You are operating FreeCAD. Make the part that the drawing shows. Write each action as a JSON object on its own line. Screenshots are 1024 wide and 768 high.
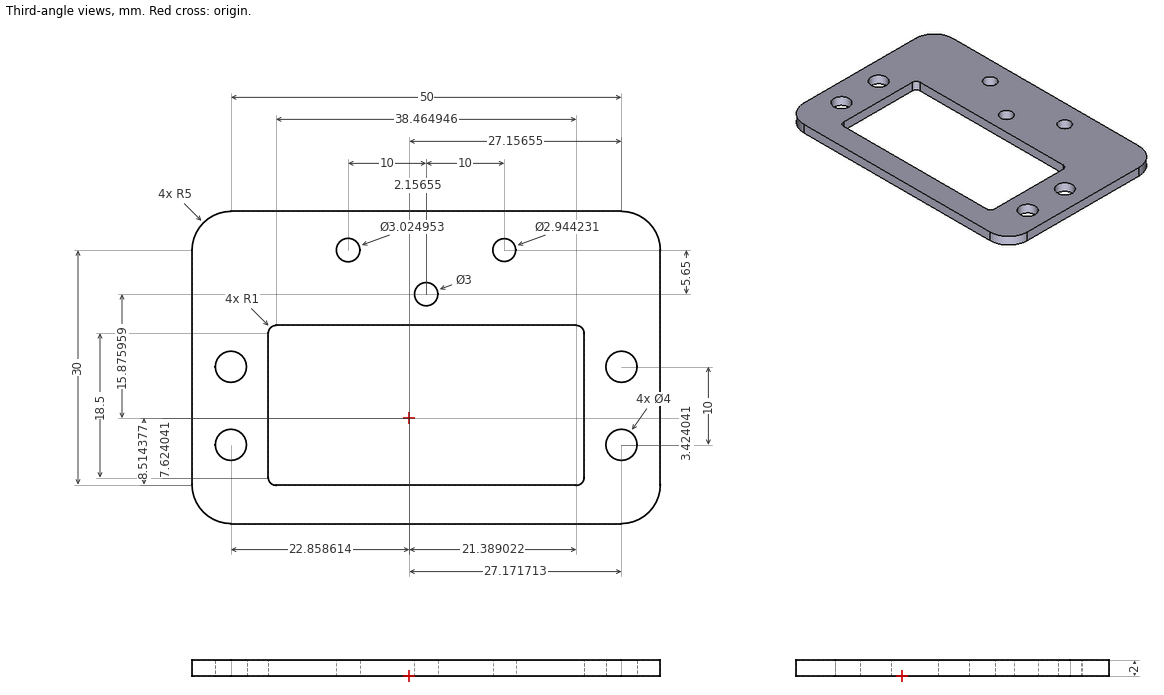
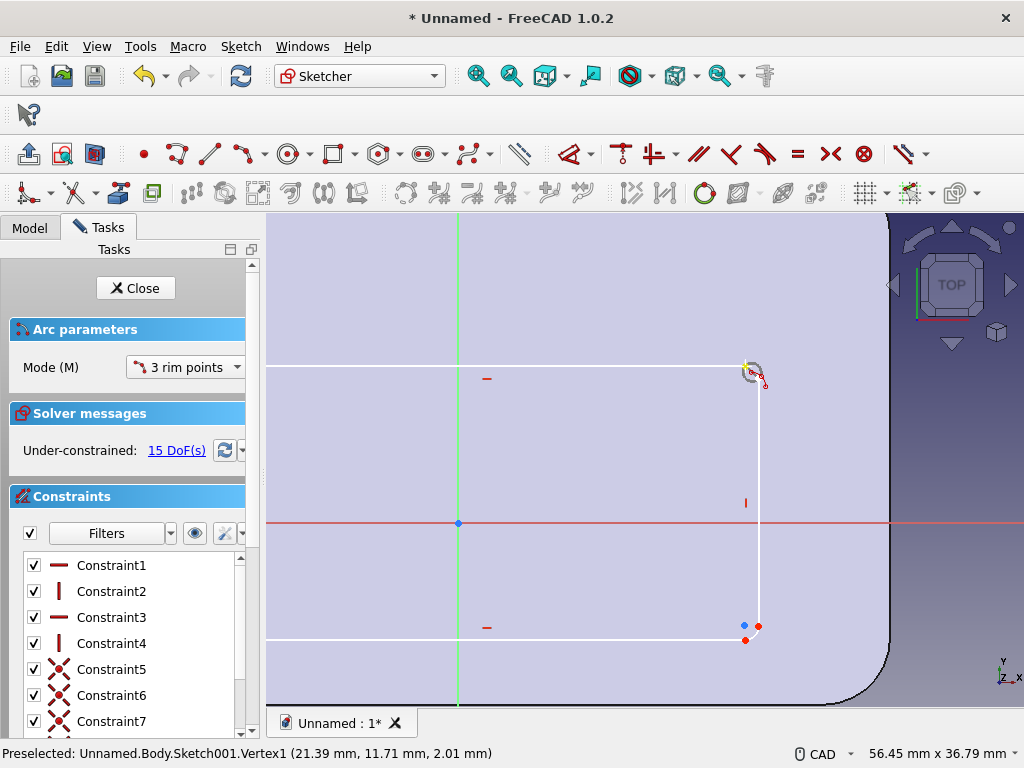
{"action": "scroll", "coordinate": [755, 368], "scroll_direction": "up", "scroll_amount": 7}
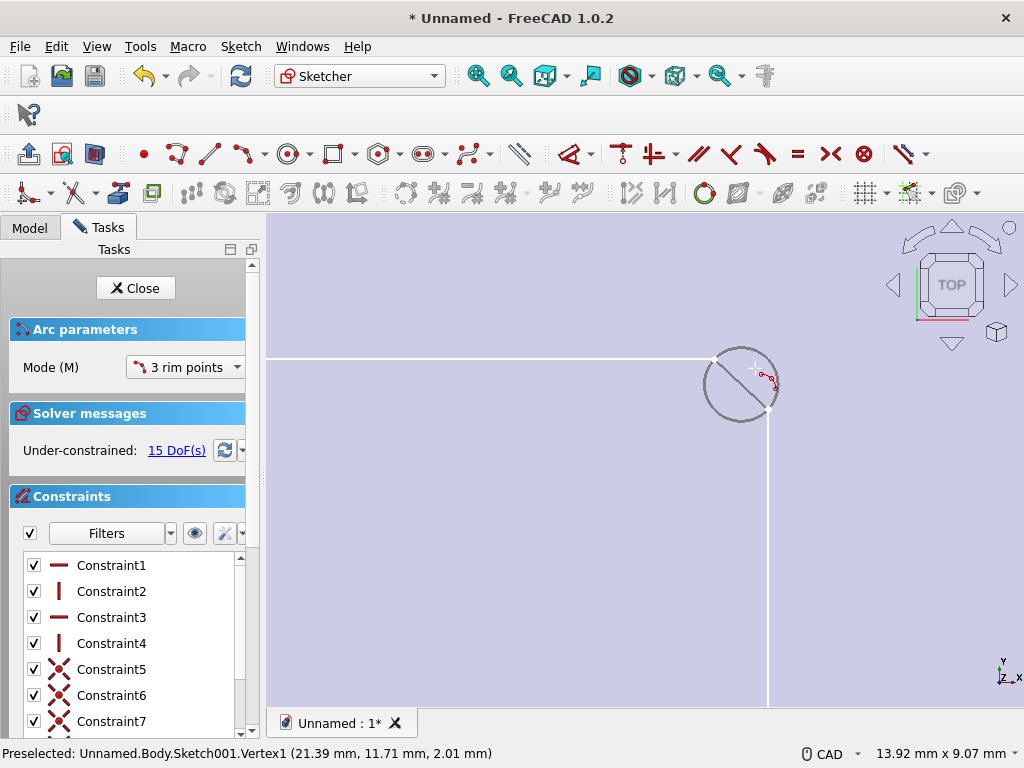
{"action": "left_click", "coordinate": [753, 366]}
{"action": "key", "text": "Escape"}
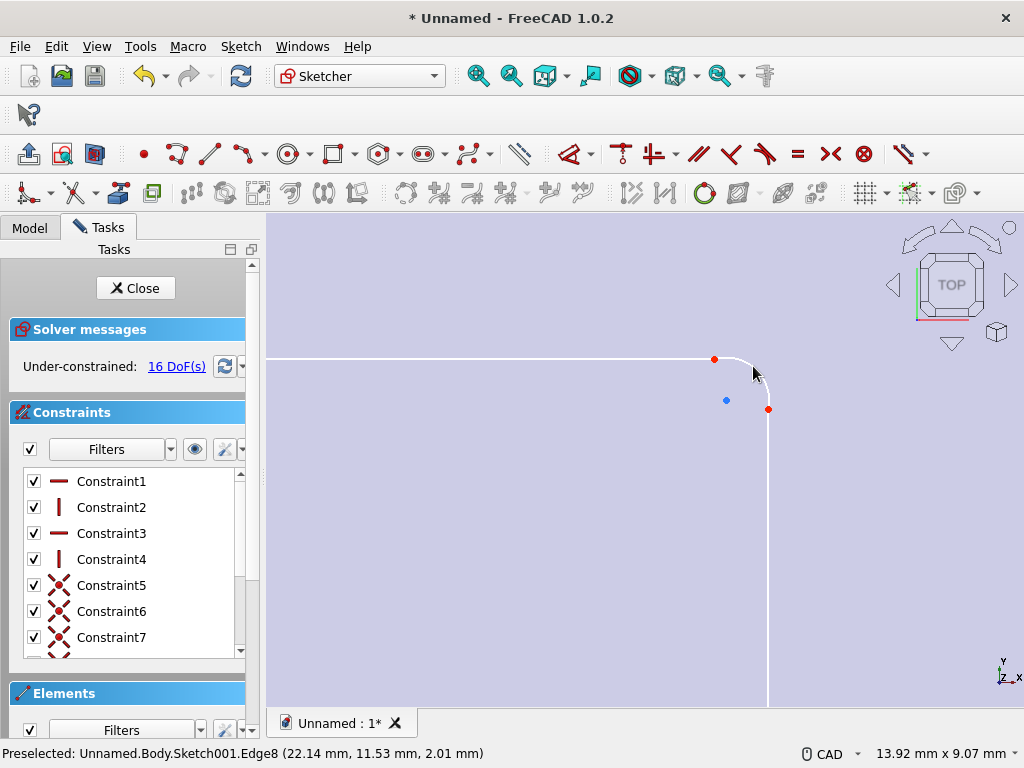
{"action": "scroll", "coordinate": [757, 371], "scroll_direction": "down", "scroll_amount": 9}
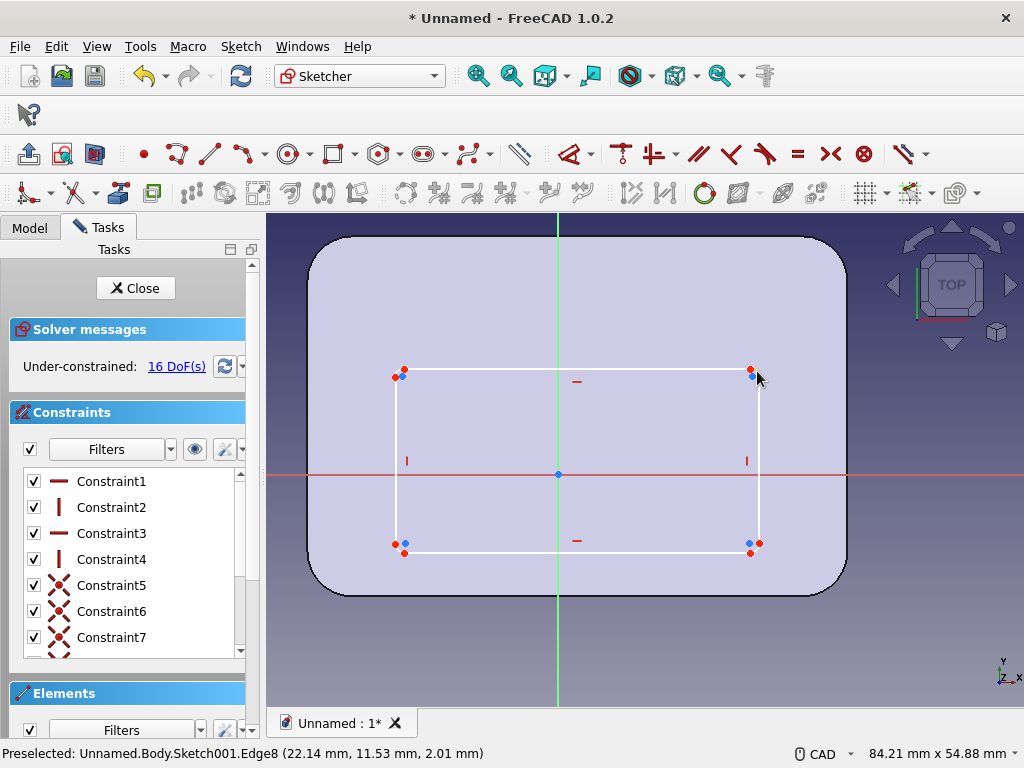
{"action": "left_click", "coordinate": [681, 369]}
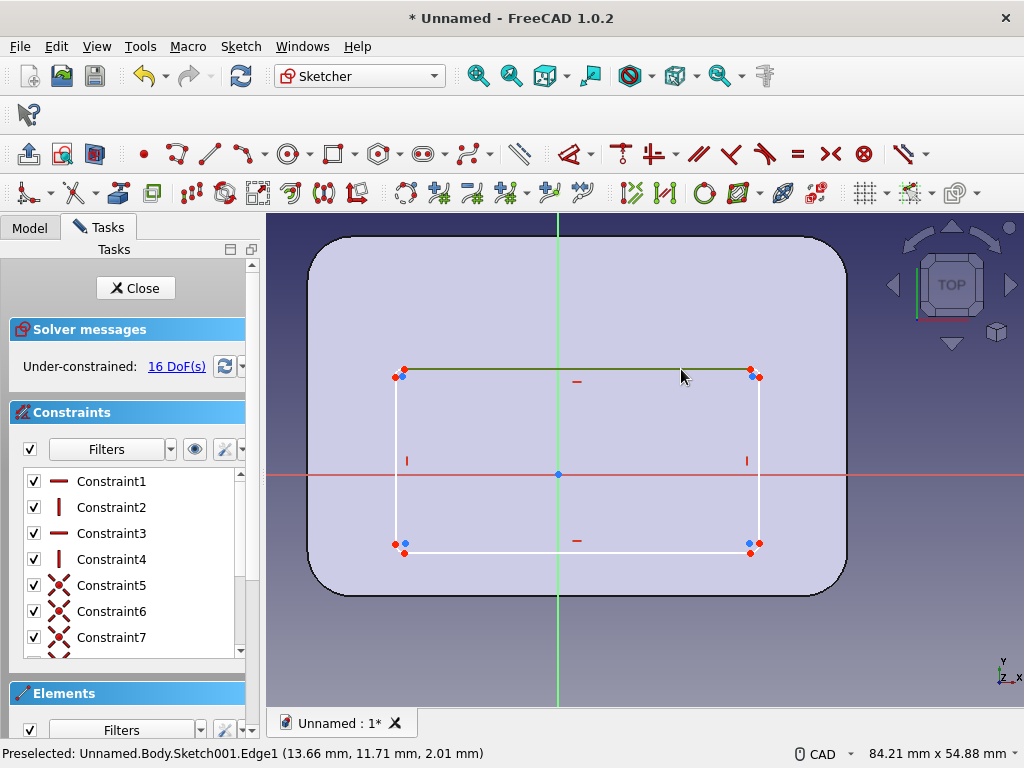
{"action": "scroll", "coordinate": [398, 371], "scroll_direction": "up", "scroll_amount": 4}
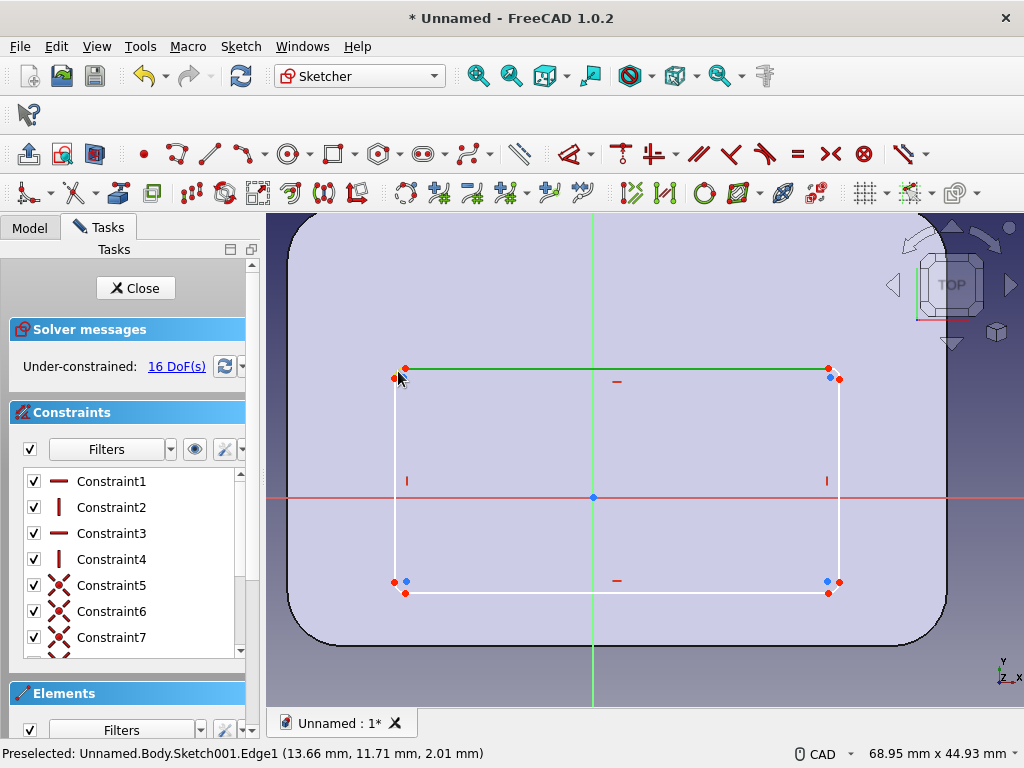
{"action": "left_click", "coordinate": [397, 370]}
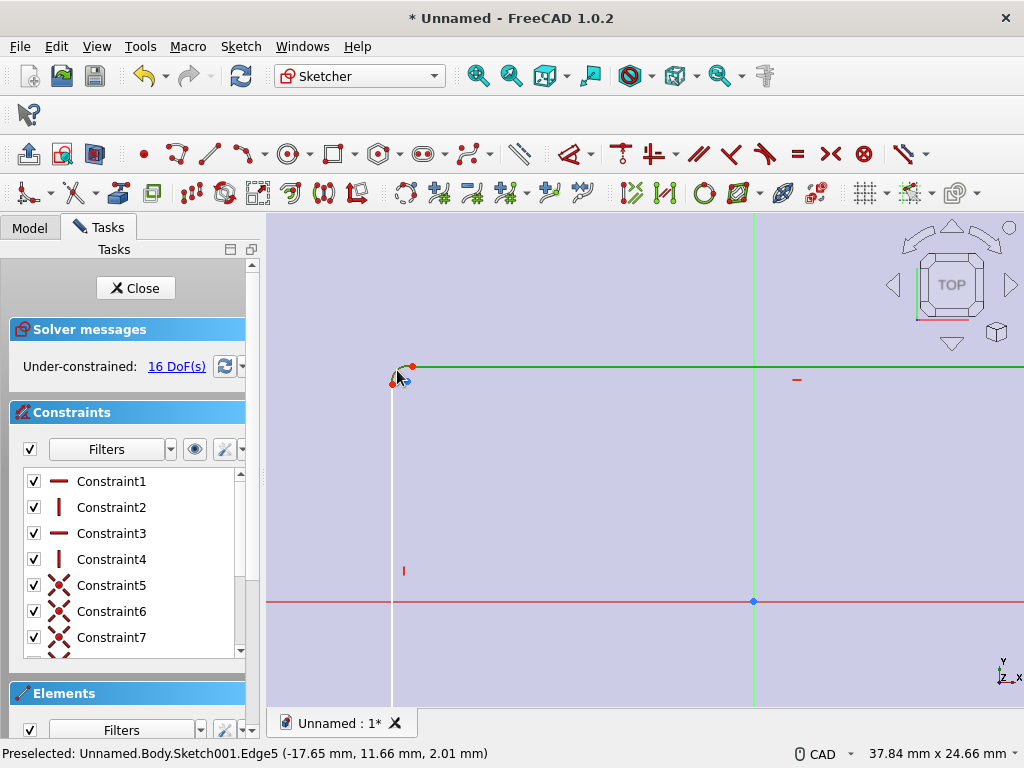
{"action": "left_click", "coordinate": [765, 154]}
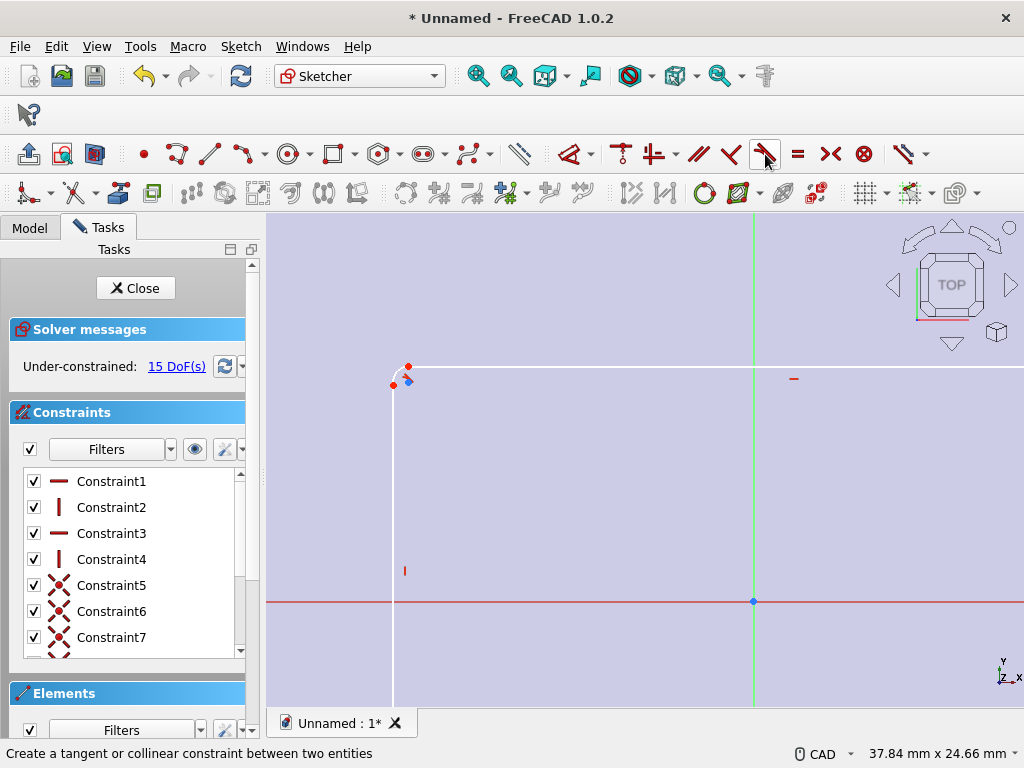
{"action": "left_click", "coordinate": [640, 367]}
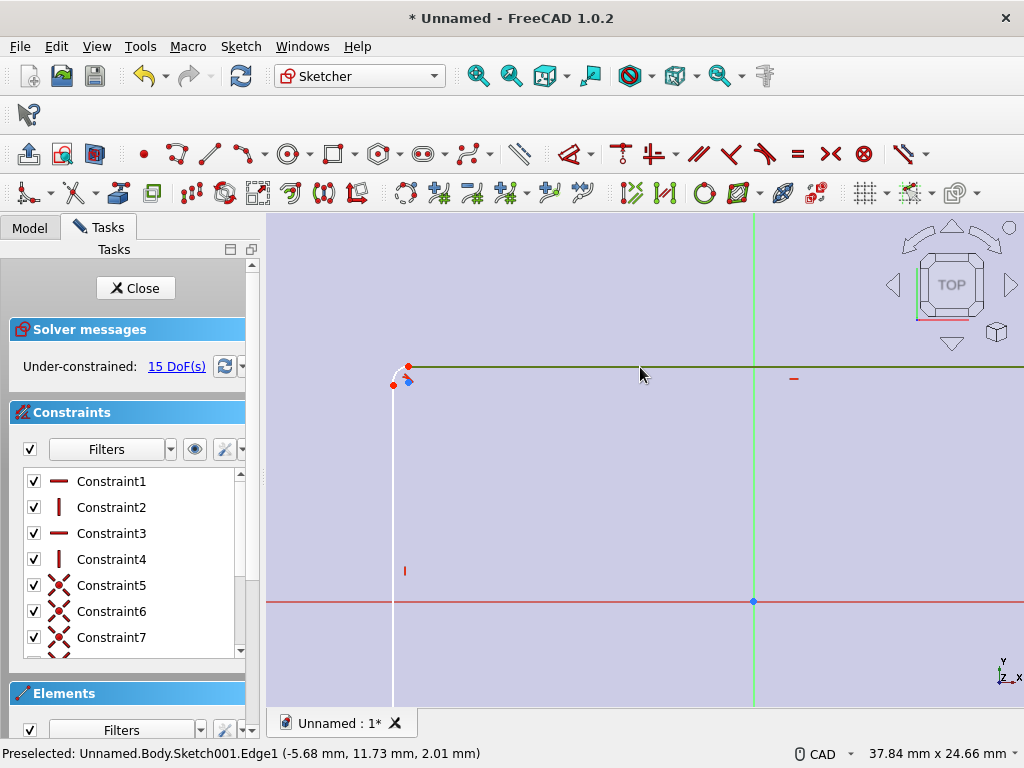
{"action": "scroll", "coordinate": [397, 371], "scroll_direction": "down", "scroll_amount": 4}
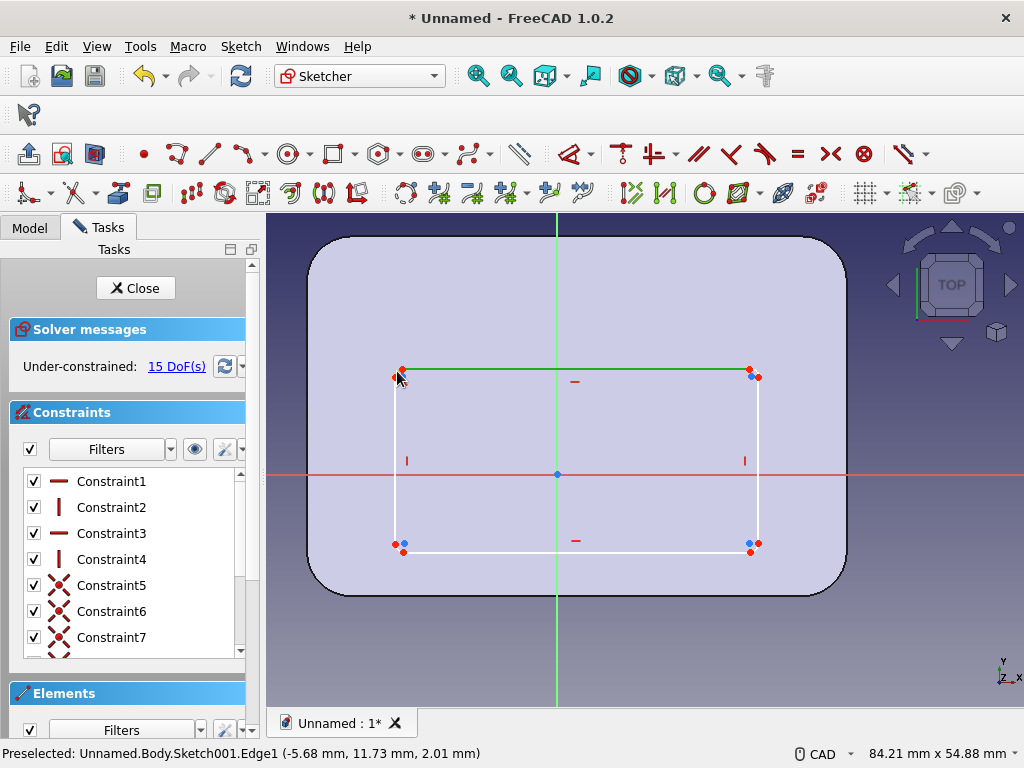
{"action": "scroll", "coordinate": [758, 373], "scroll_direction": "up", "scroll_amount": 6}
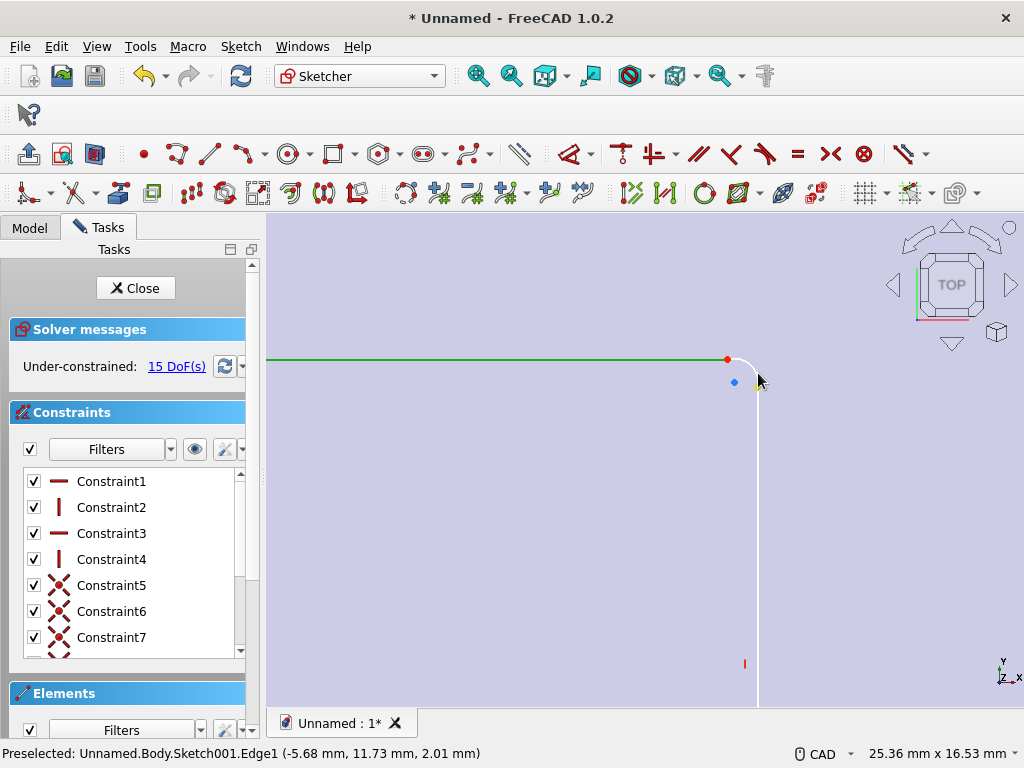
{"action": "left_click", "coordinate": [756, 373]}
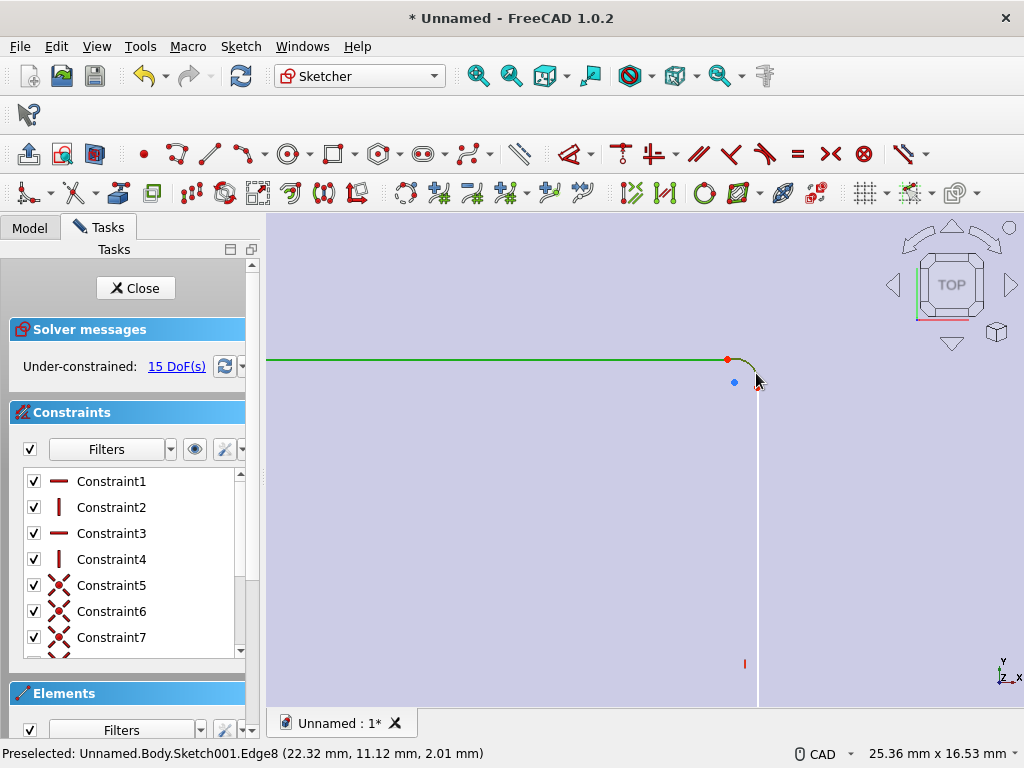
{"action": "left_click", "coordinate": [765, 154]}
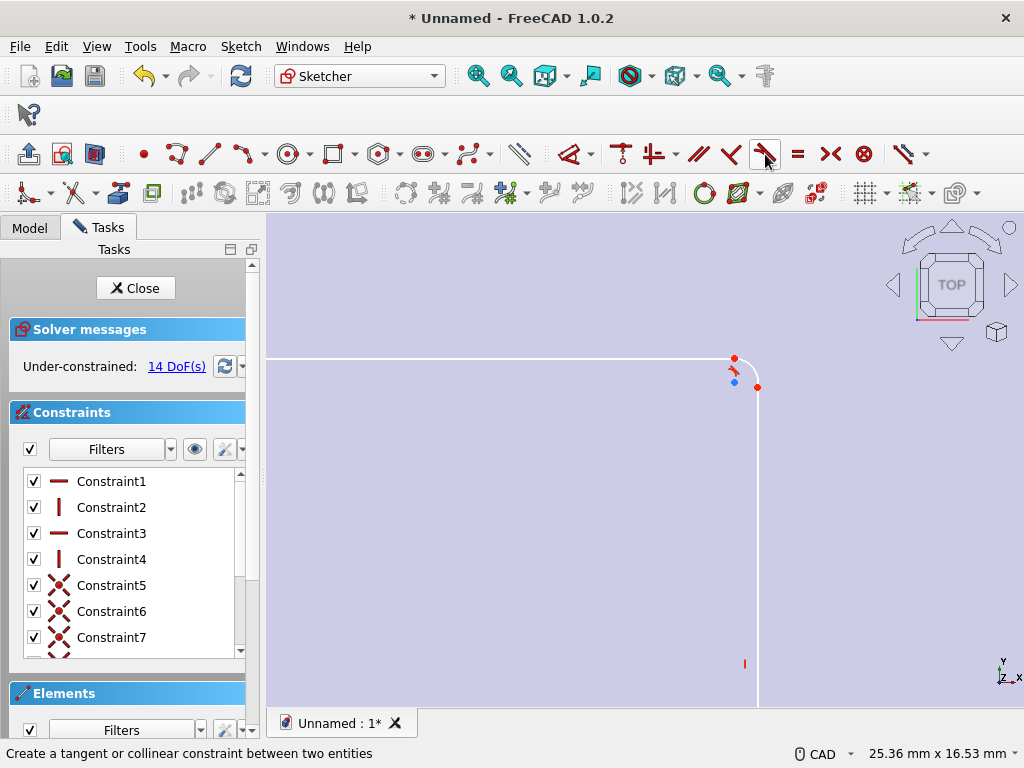
{"action": "scroll", "coordinate": [758, 373], "scroll_direction": "down", "scroll_amount": 6}